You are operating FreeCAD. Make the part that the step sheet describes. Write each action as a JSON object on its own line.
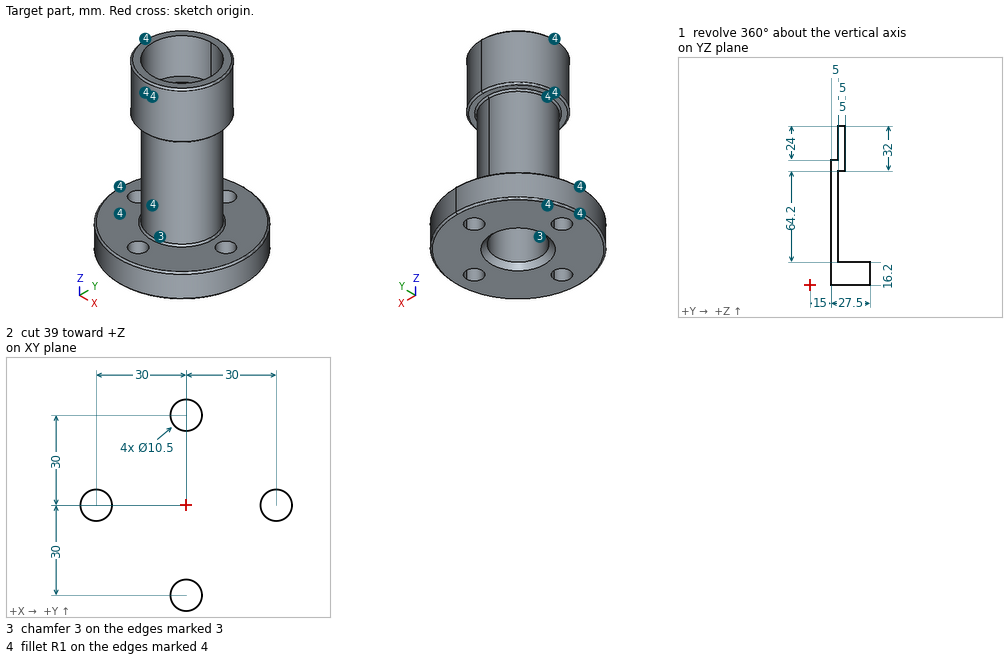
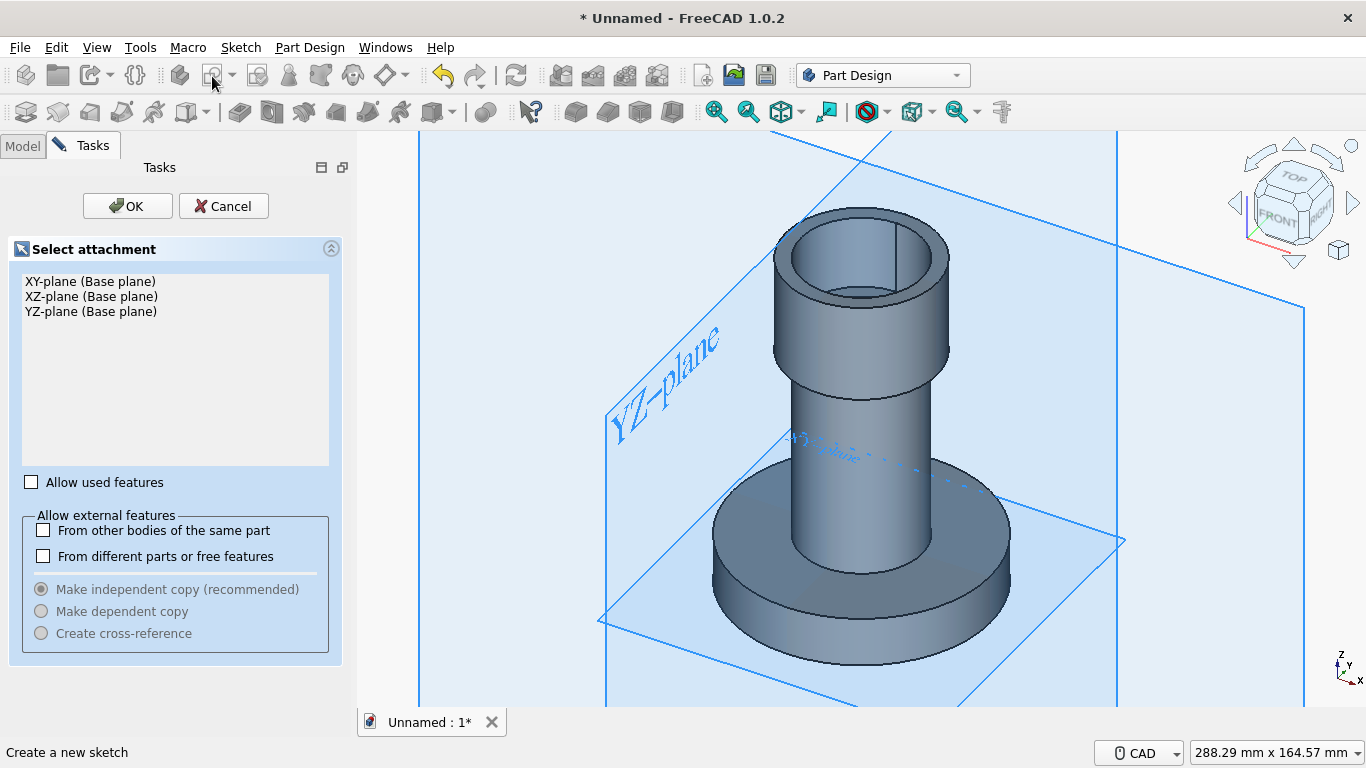
{"action": "left_click", "coordinate": [82, 282]}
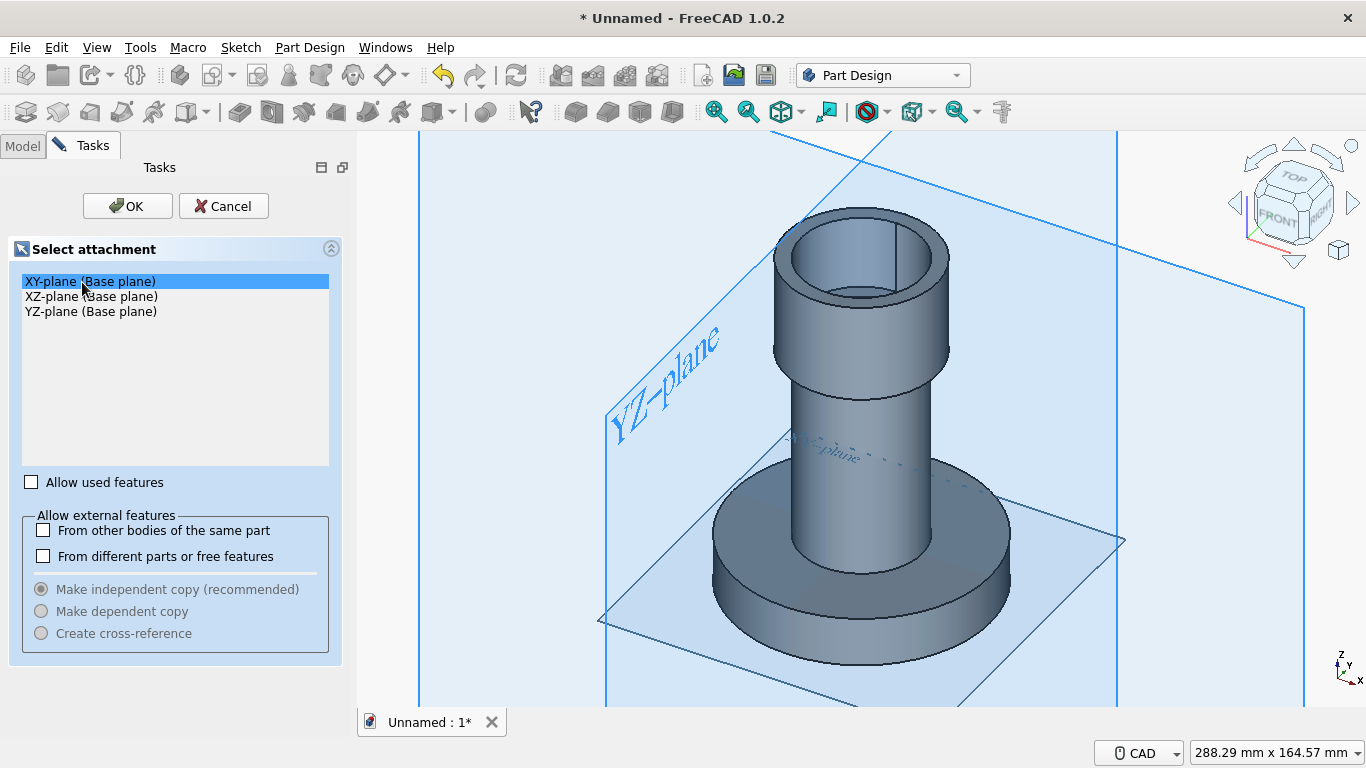
{"action": "left_click", "coordinate": [128, 206]}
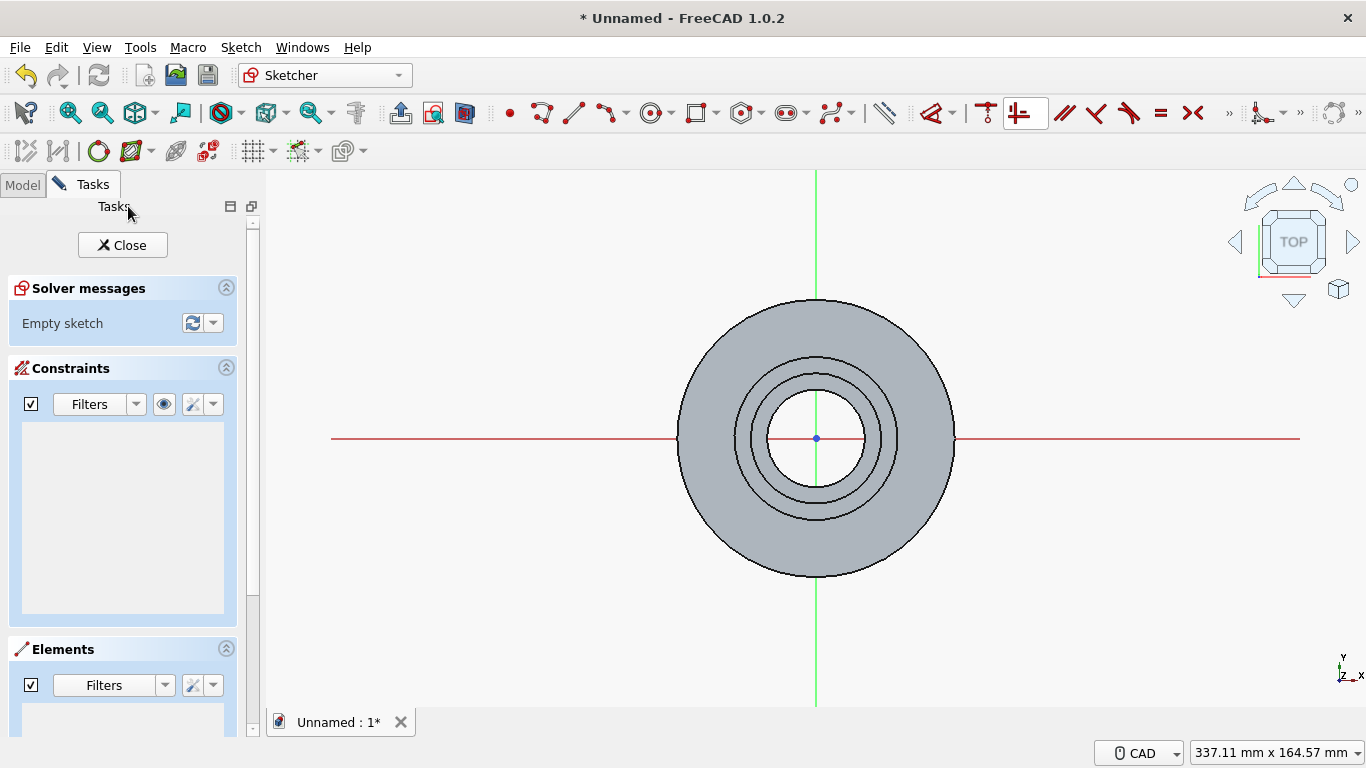
{"action": "left_click", "coordinate": [466, 114]}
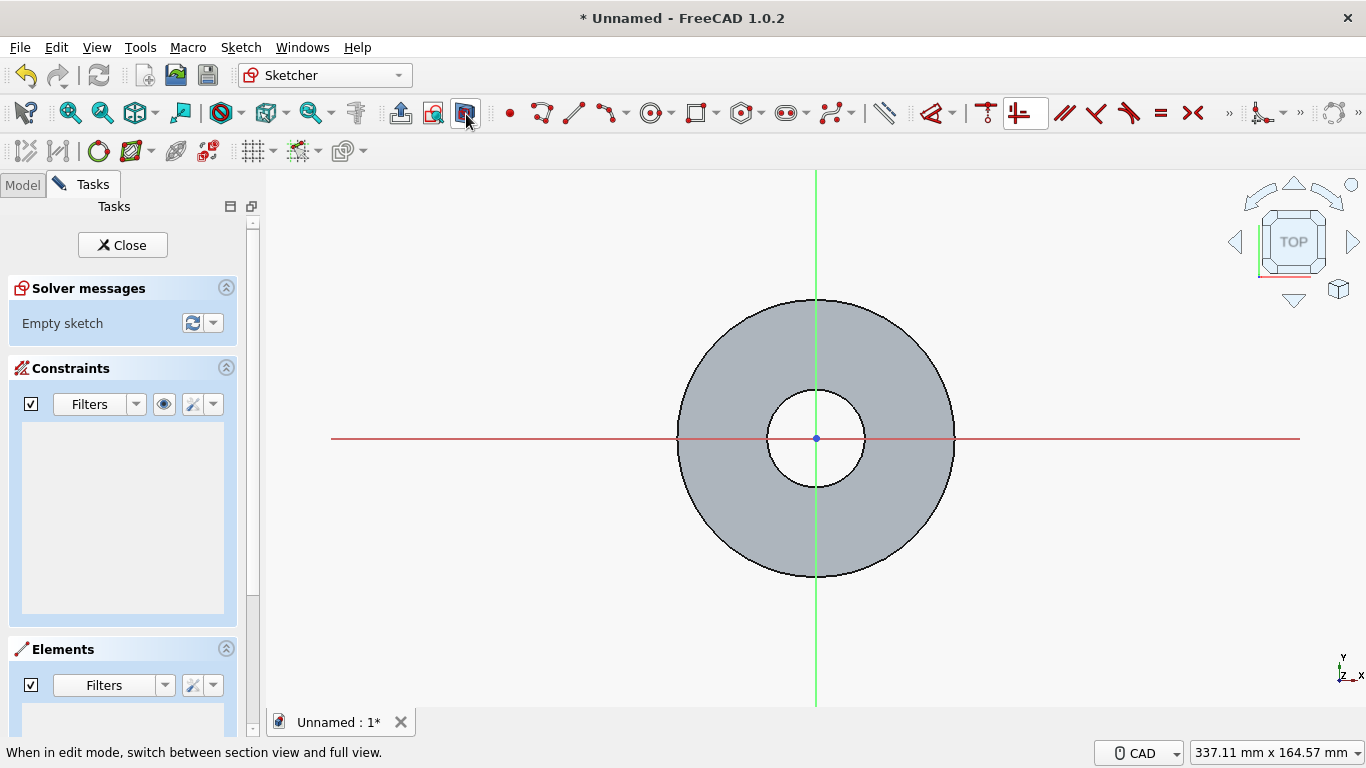
{"action": "scroll", "coordinate": [955, 439], "scroll_direction": "up", "scroll_amount": 2}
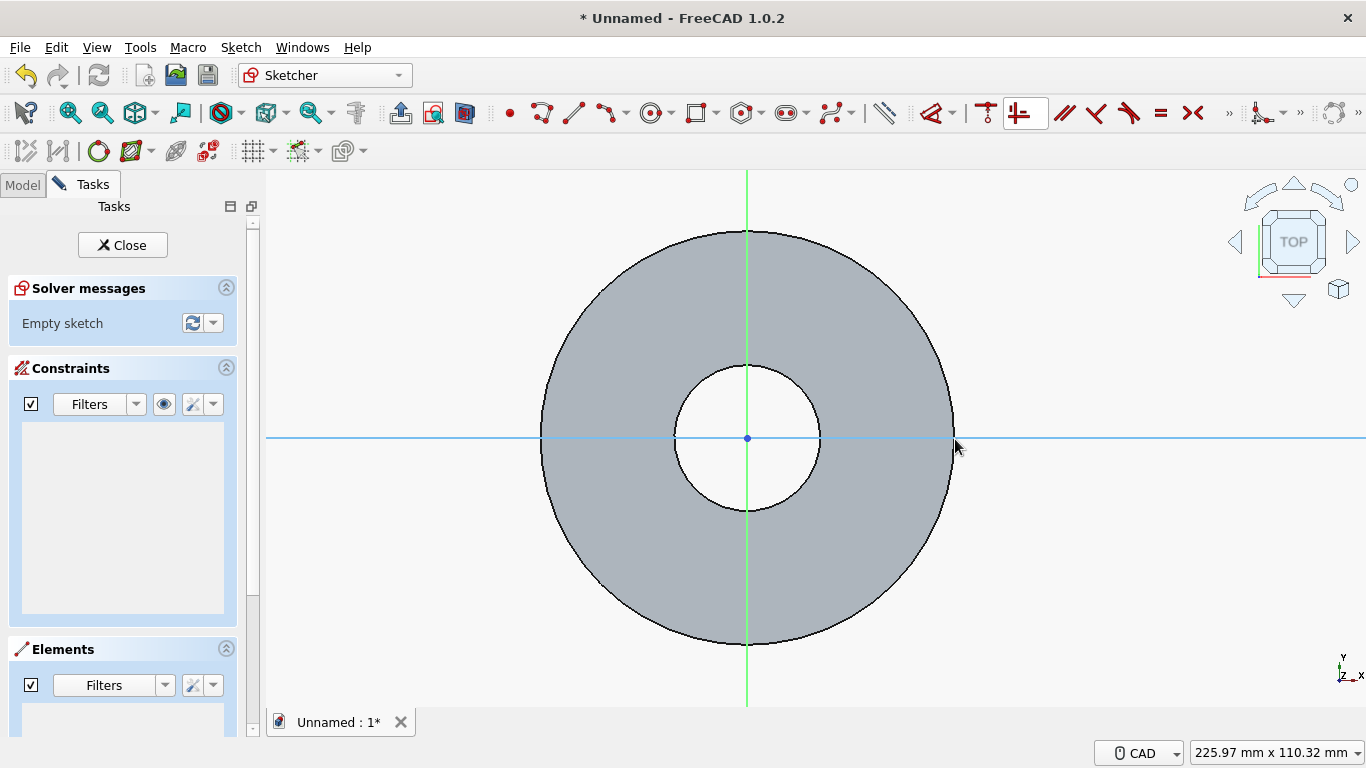
{"action": "left_click", "coordinate": [652, 114]}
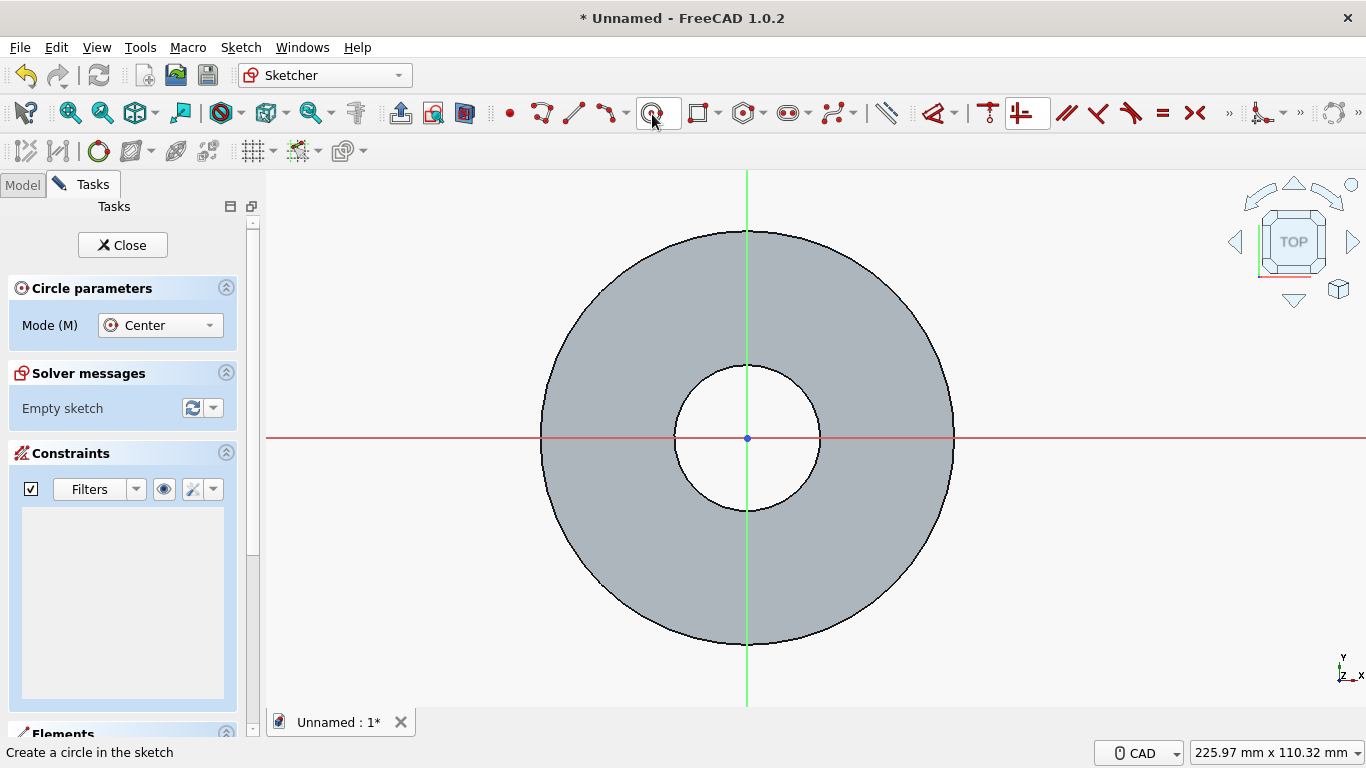
{"action": "left_click", "coordinate": [747, 292]}
{"action": "left_click", "coordinate": [765, 274]}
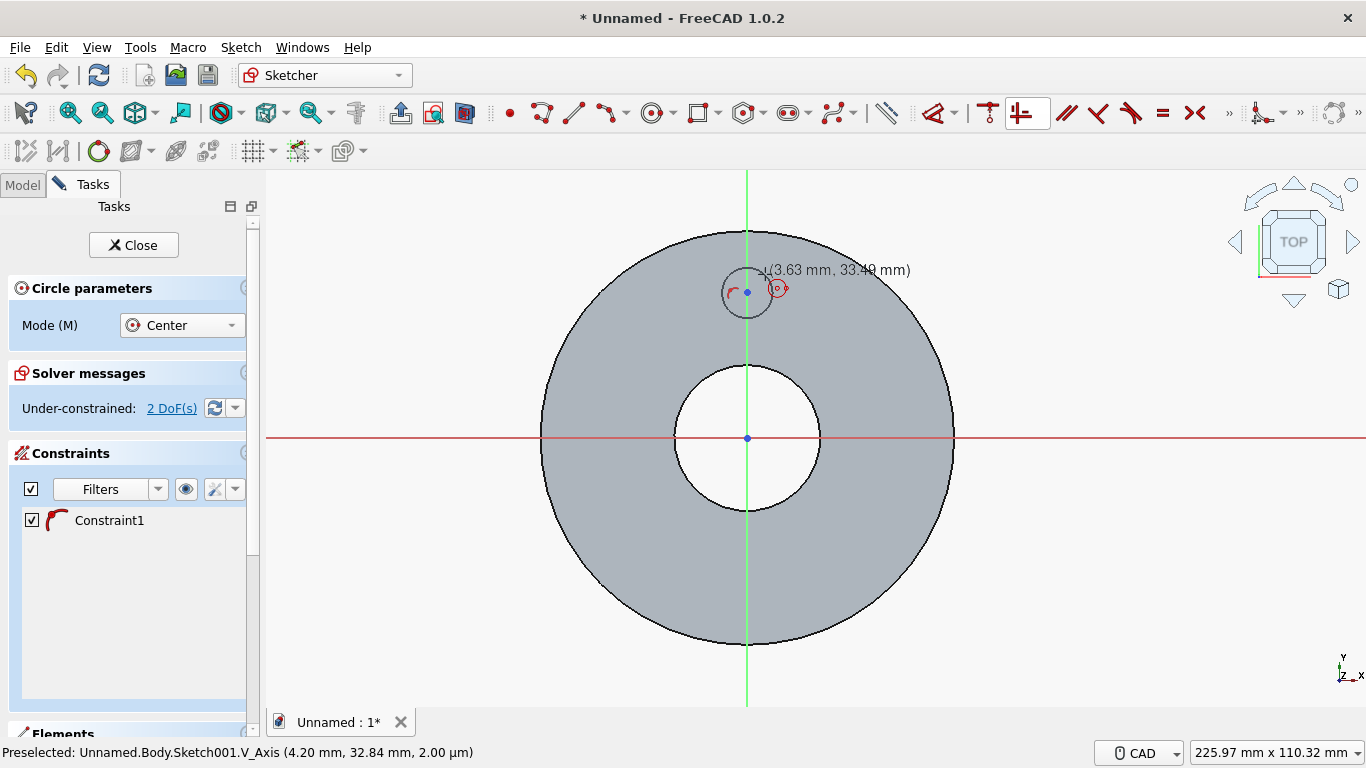
{"action": "left_click", "coordinate": [601, 438]}
{"action": "left_click", "coordinate": [619, 420]}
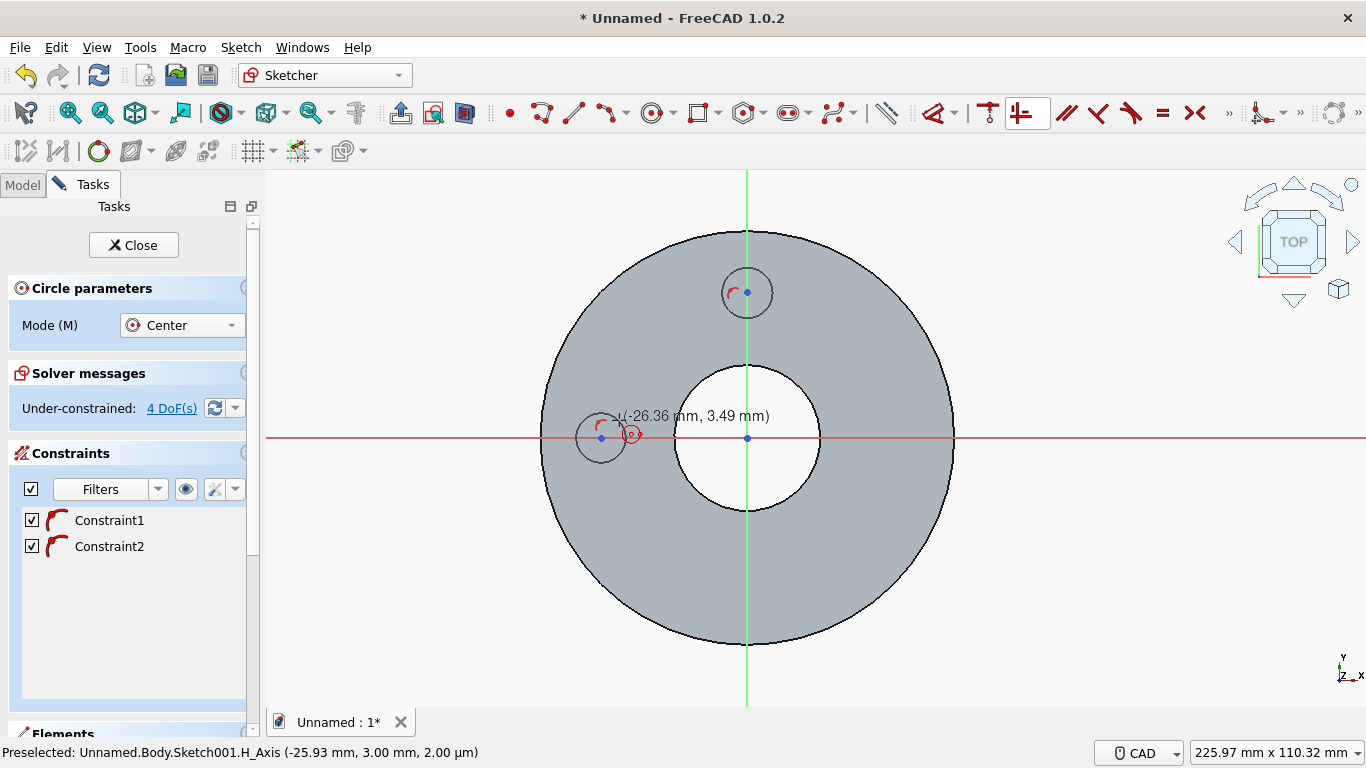
{"action": "left_click", "coordinate": [747, 584]}
{"action": "left_click", "coordinate": [765, 566]}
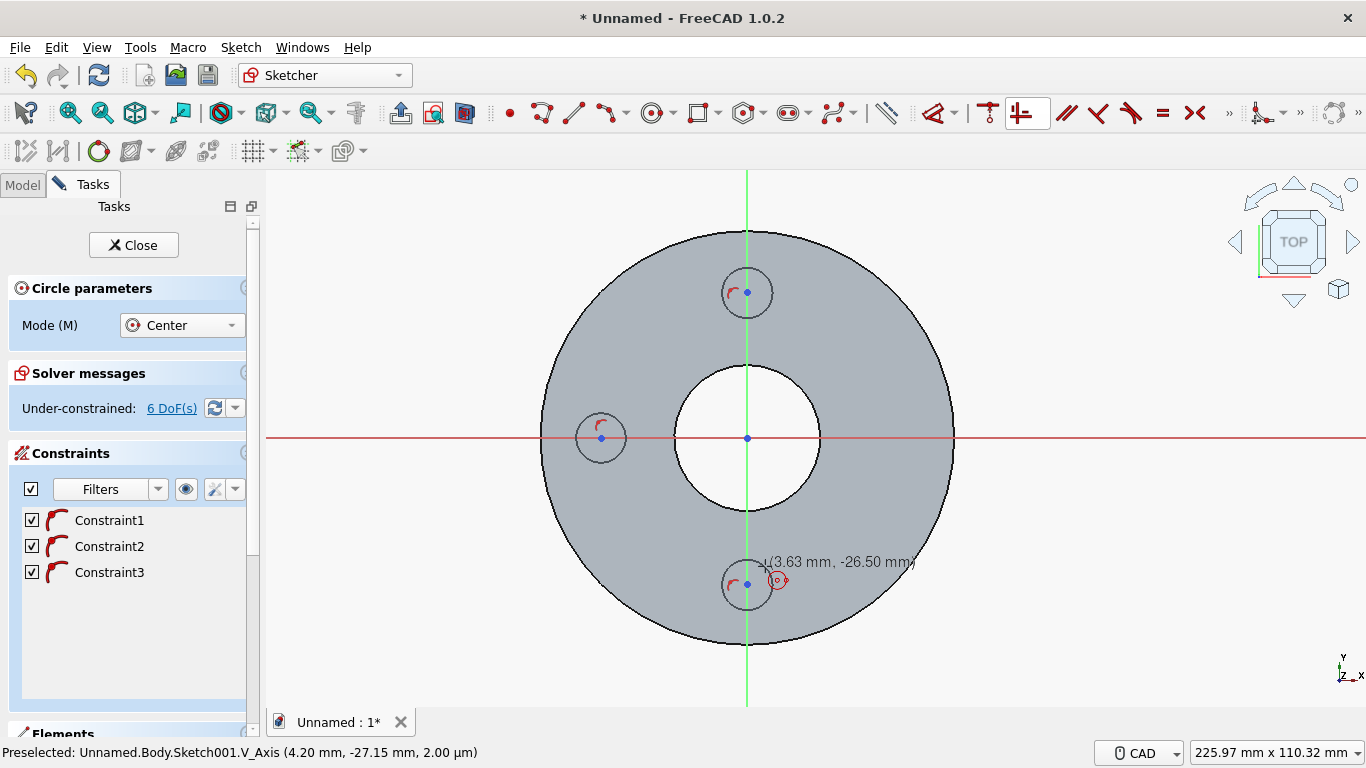
{"action": "left_click", "coordinate": [893, 438]}
{"action": "left_click", "coordinate": [911, 420]}
{"action": "key", "text": "Escape"}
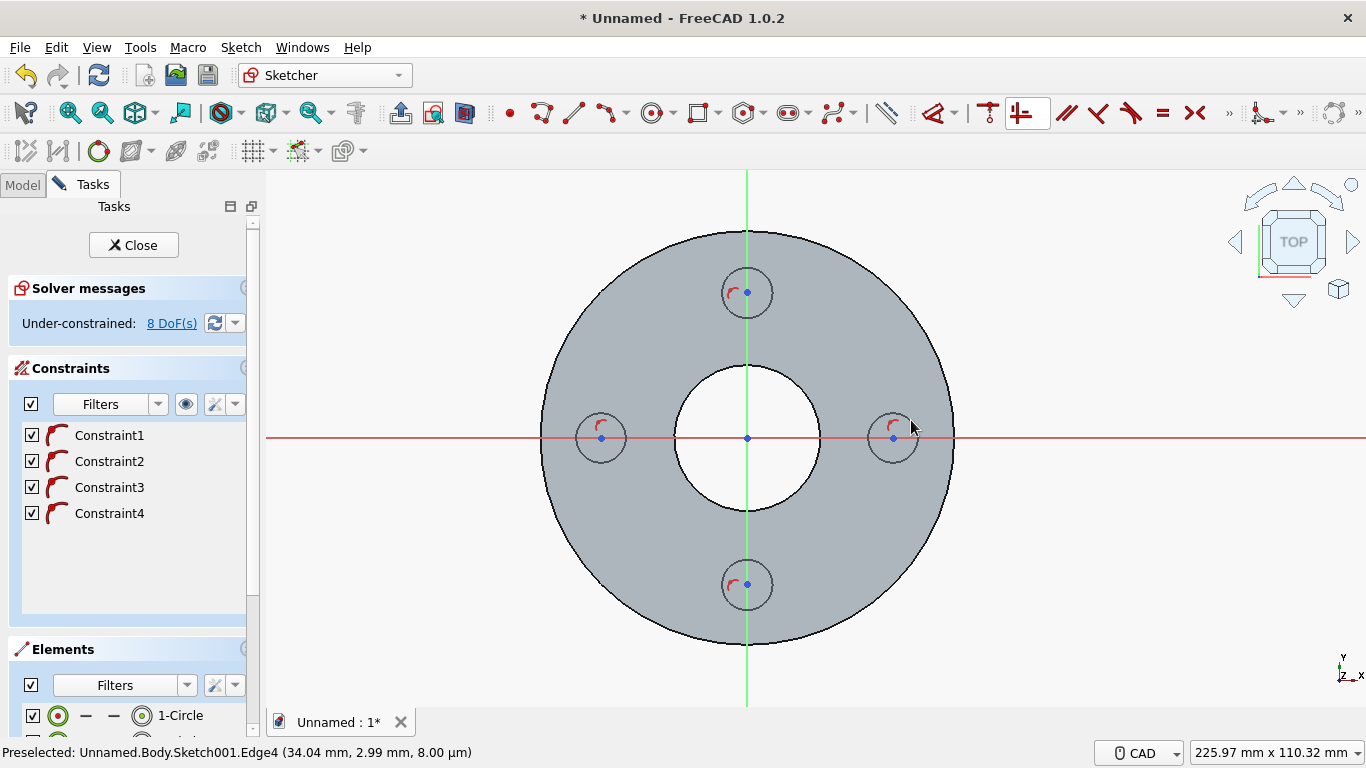
{"action": "left_click", "coordinate": [765, 275]}